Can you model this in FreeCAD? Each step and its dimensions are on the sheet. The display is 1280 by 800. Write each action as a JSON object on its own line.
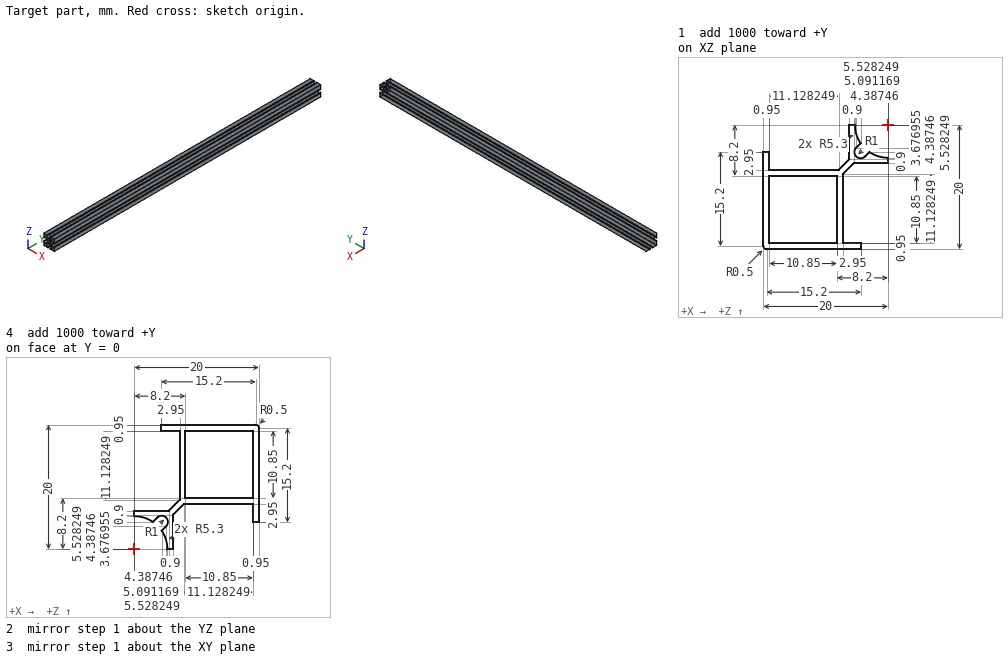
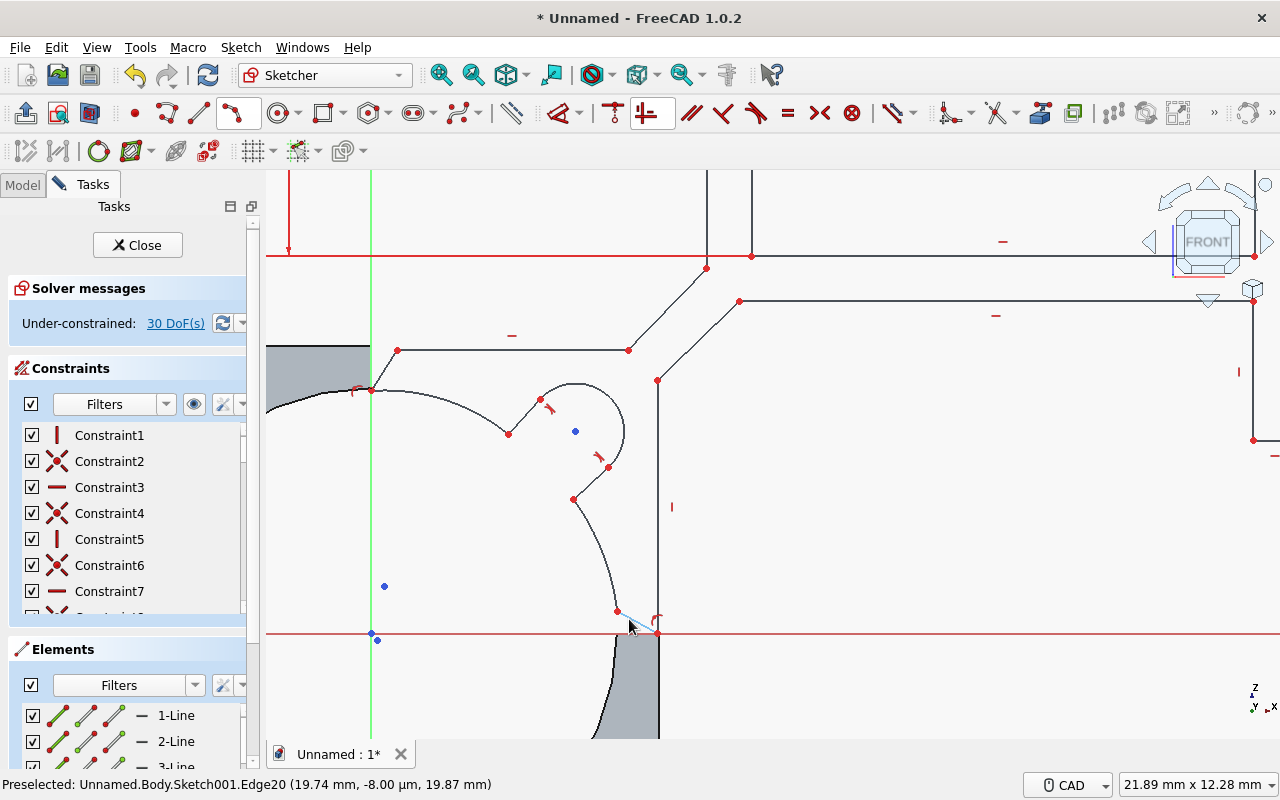
{"action": "left_click", "coordinate": [629, 618]}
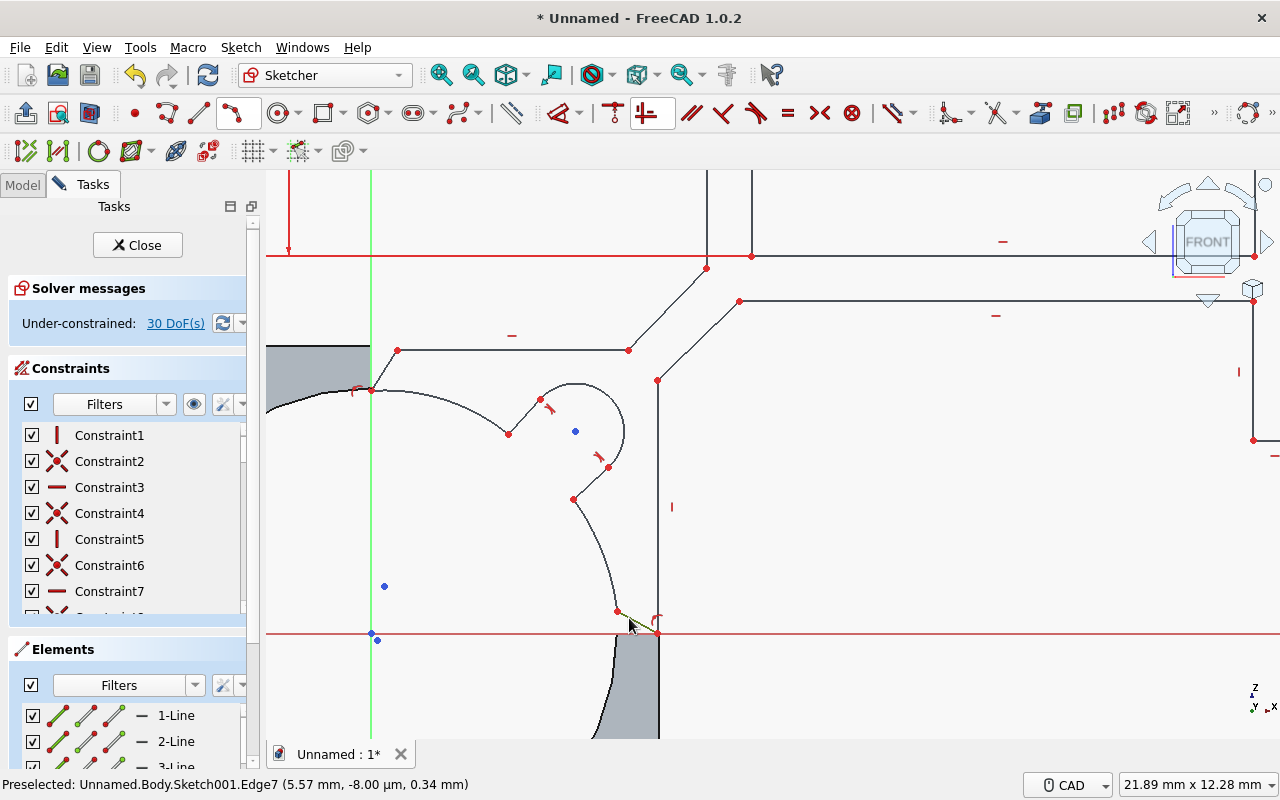
{"action": "key", "text": "h"}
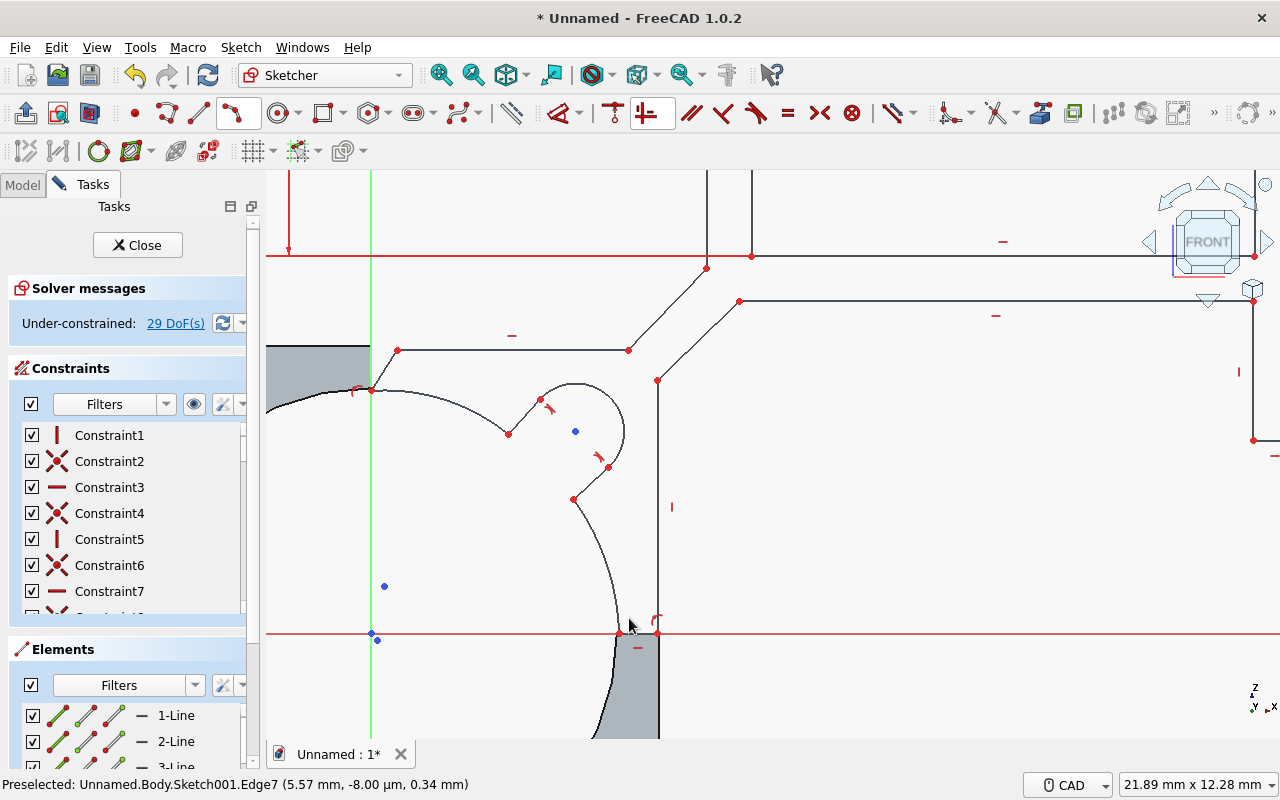
{"action": "left_click", "coordinate": [389, 362]}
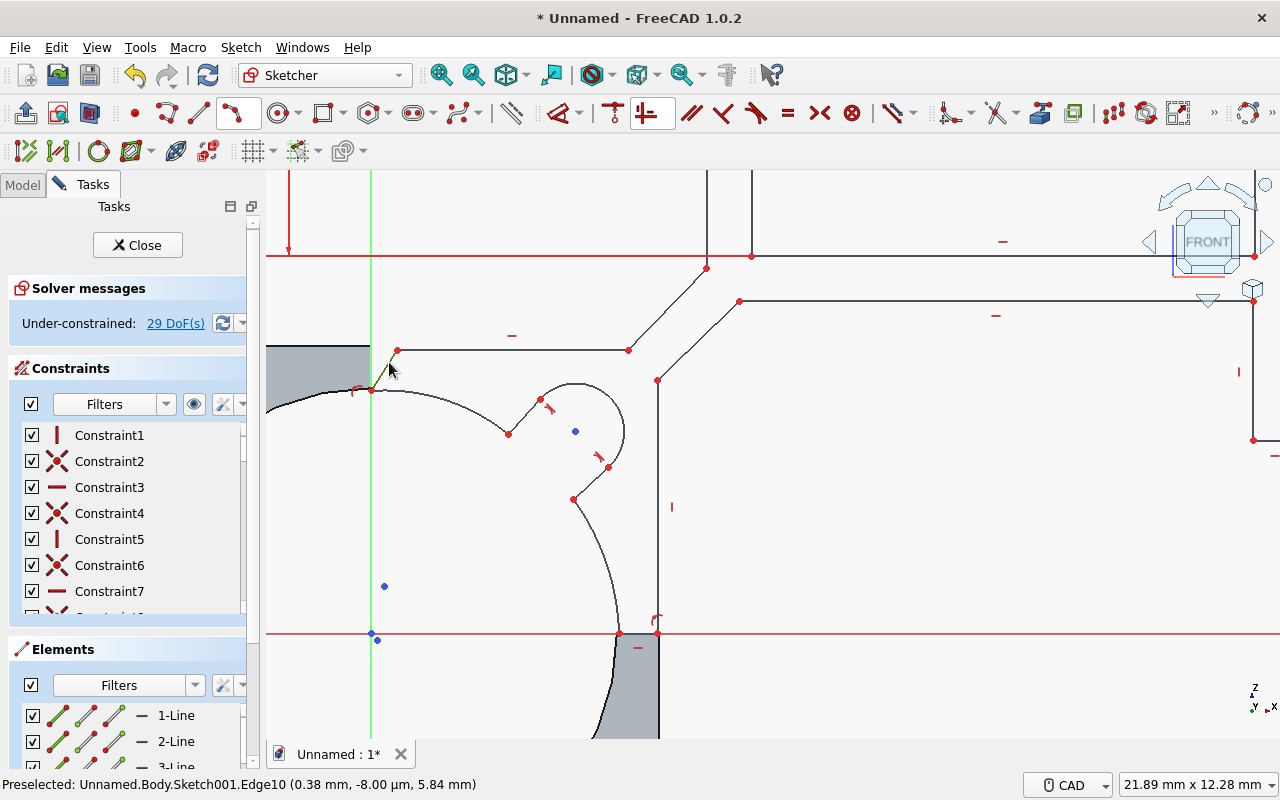
{"action": "left_click", "coordinate": [670, 114]}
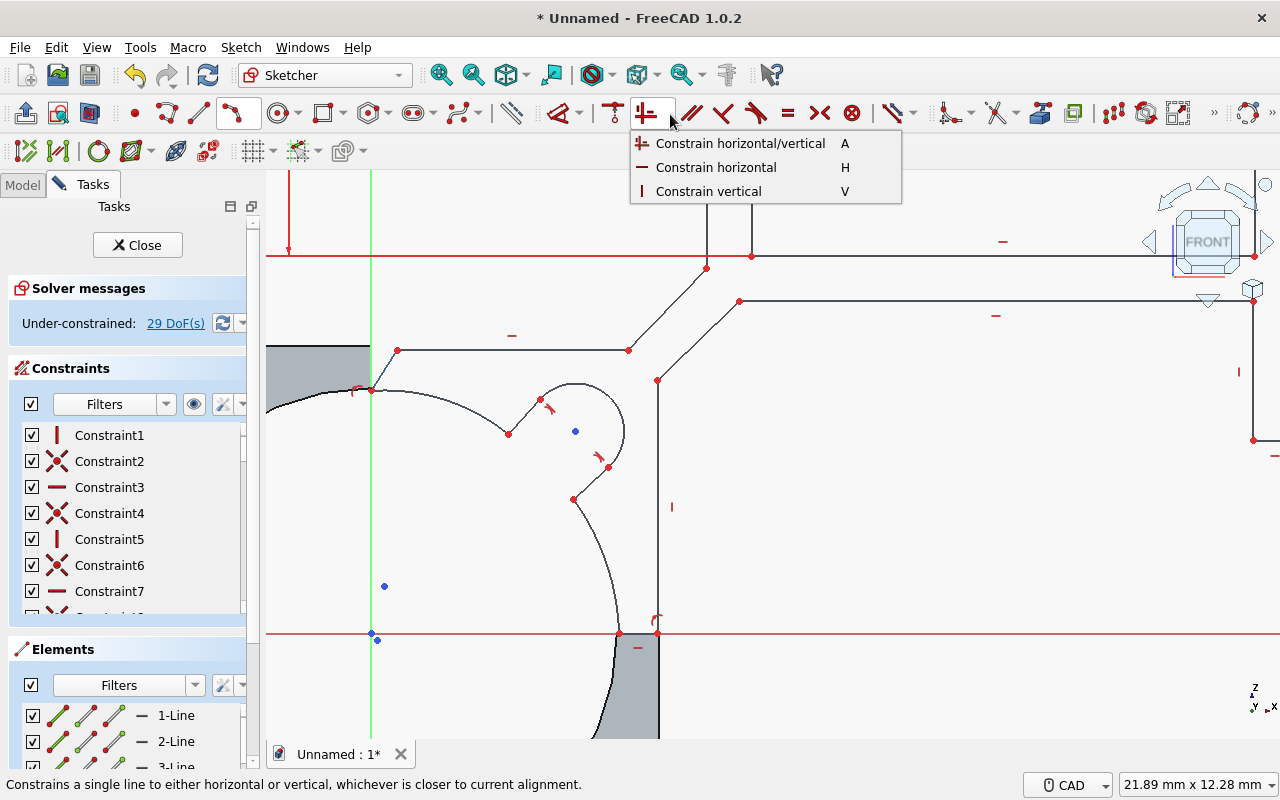
{"action": "left_click", "coordinate": [766, 191]}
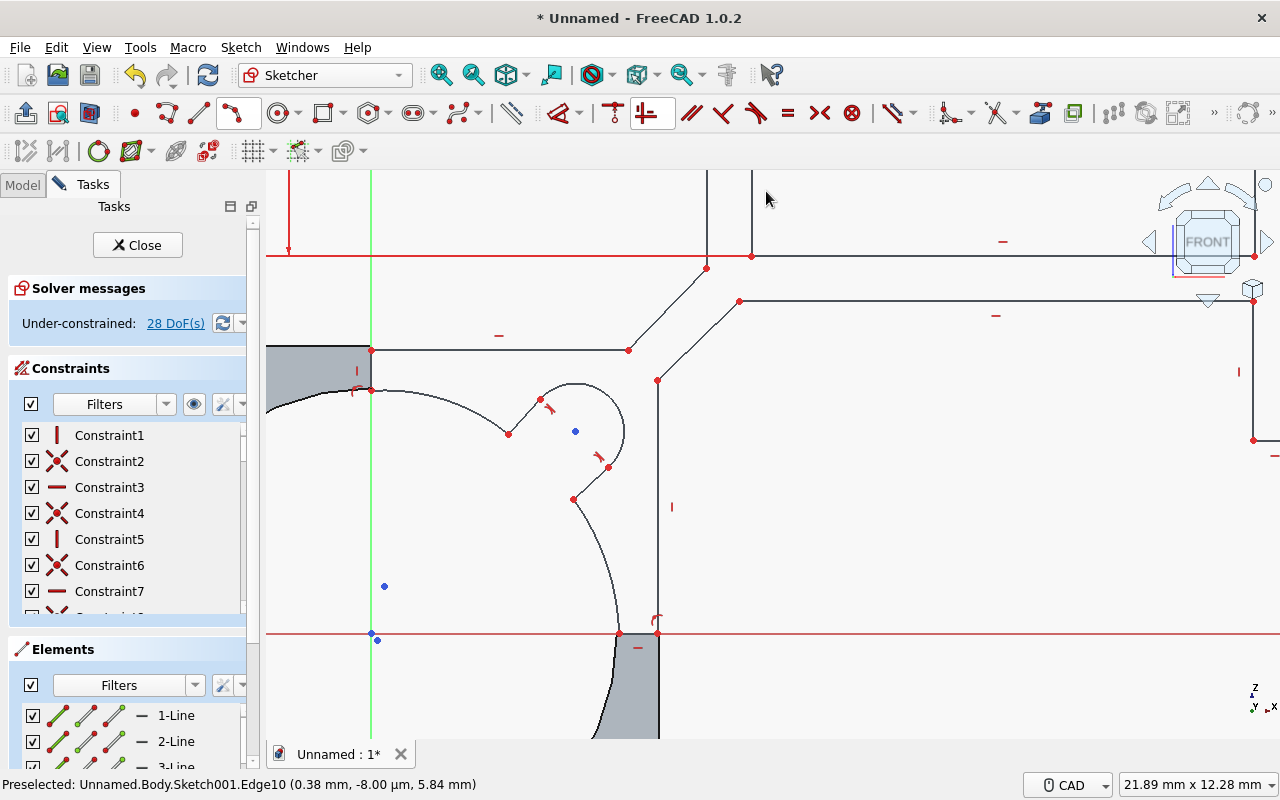
{"action": "scroll", "coordinate": [629, 620], "scroll_direction": "down", "scroll_amount": 5}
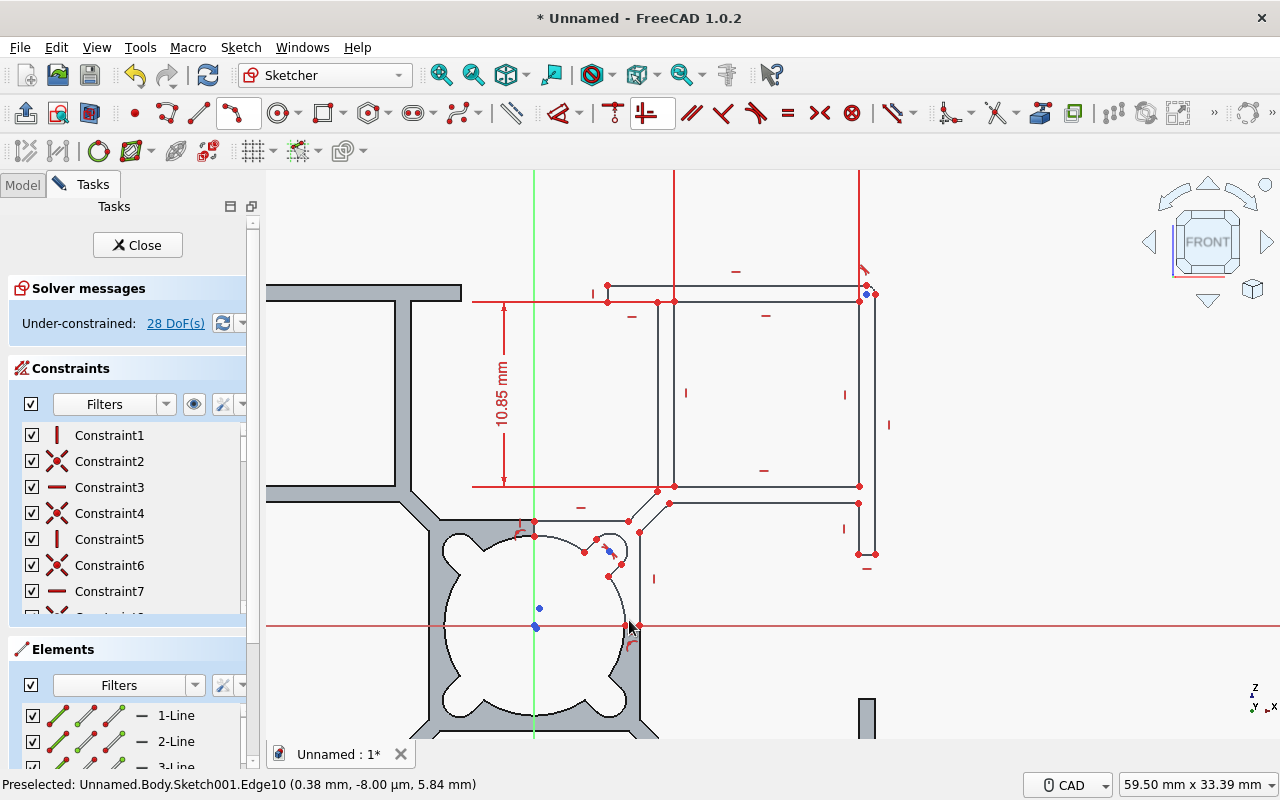
{"action": "left_click", "coordinate": [624, 610]}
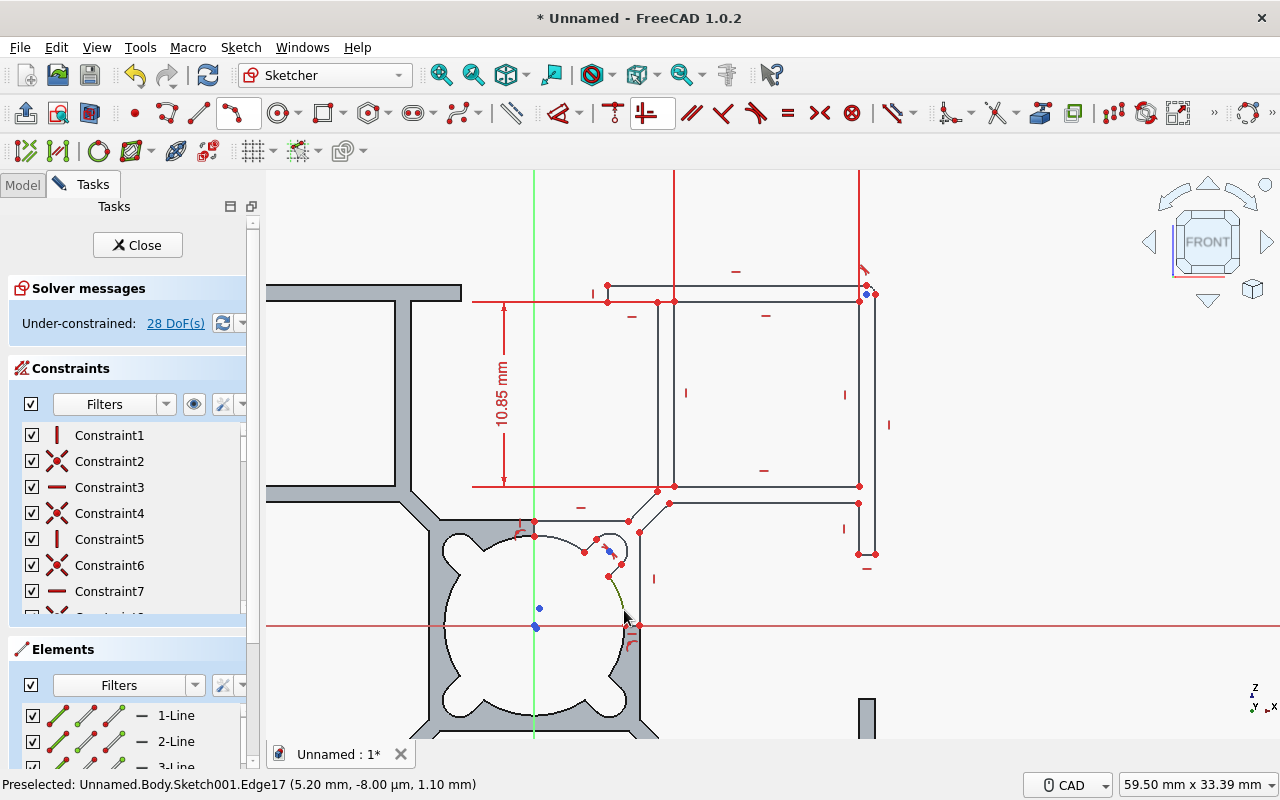
{"action": "left_click", "coordinate": [571, 543]}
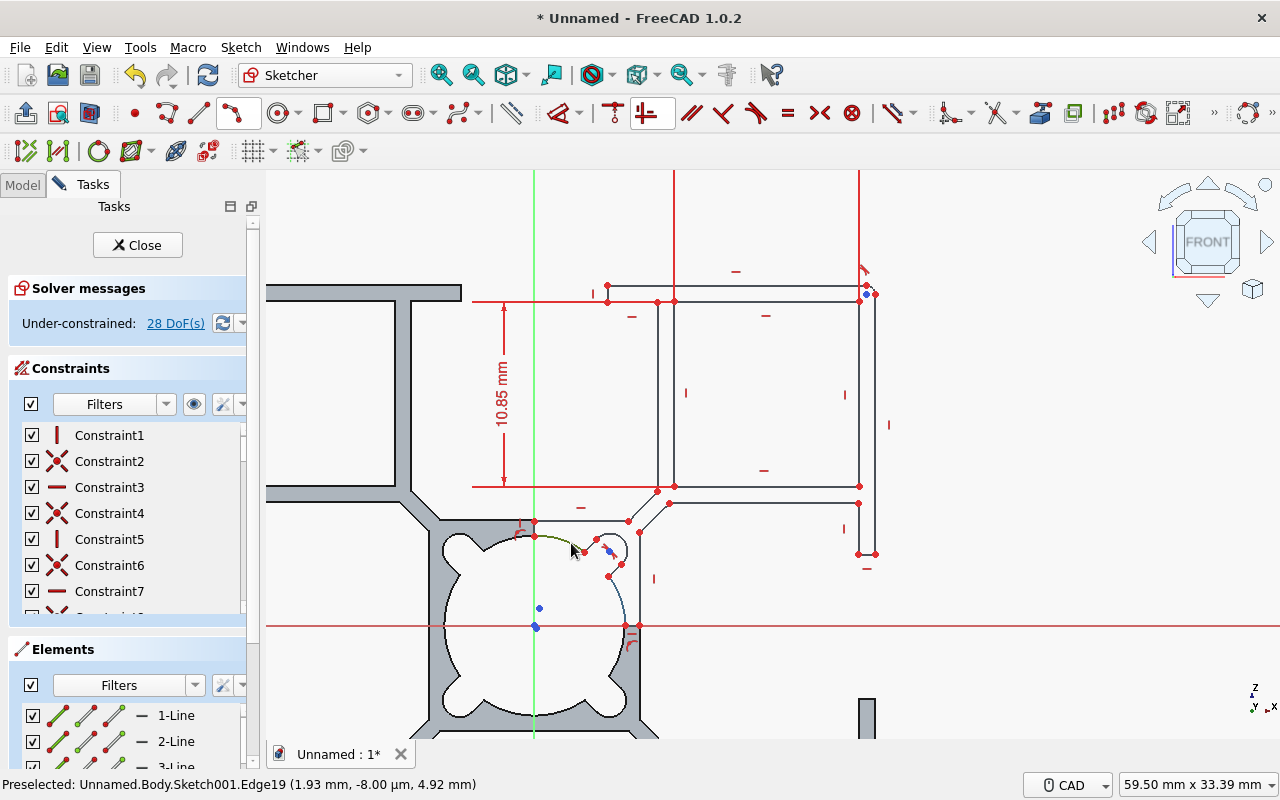
{"action": "left_click", "coordinate": [614, 114]}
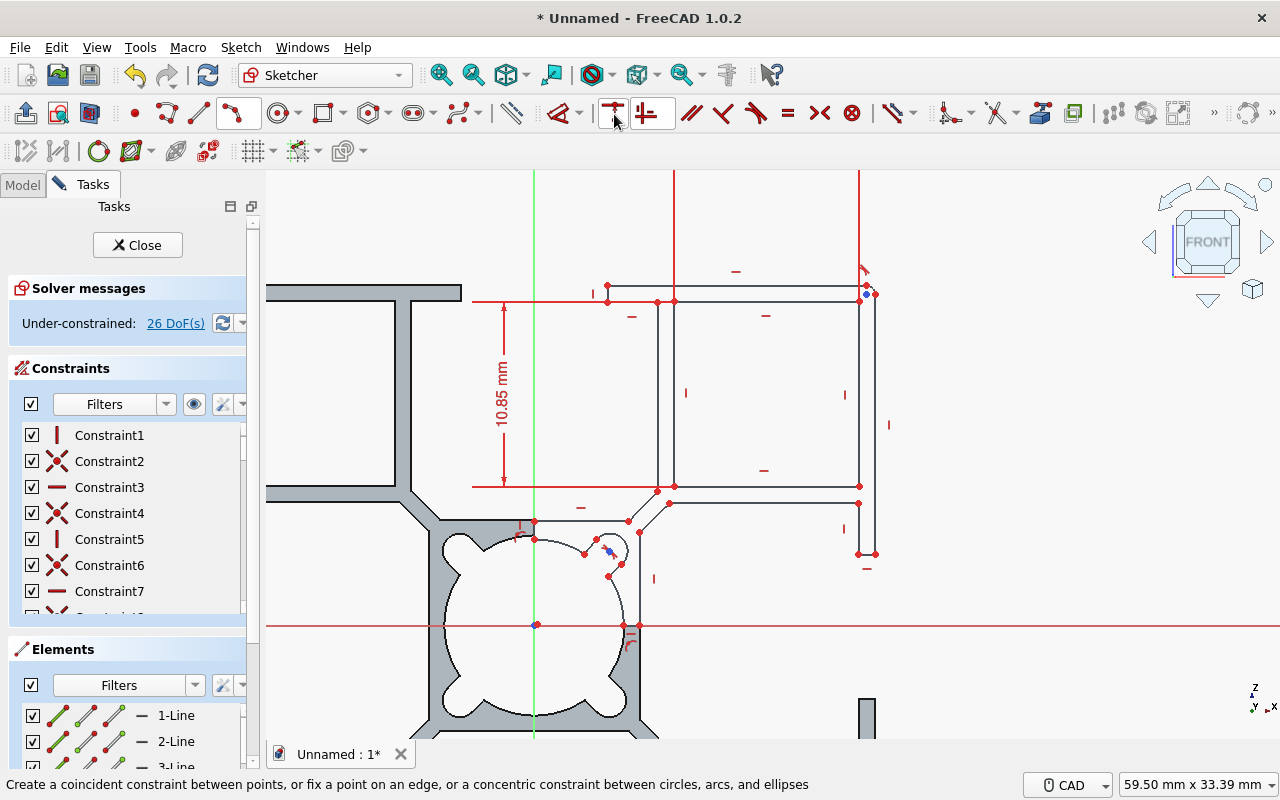
{"action": "scroll", "coordinate": [536, 625], "scroll_direction": "up", "scroll_amount": 8}